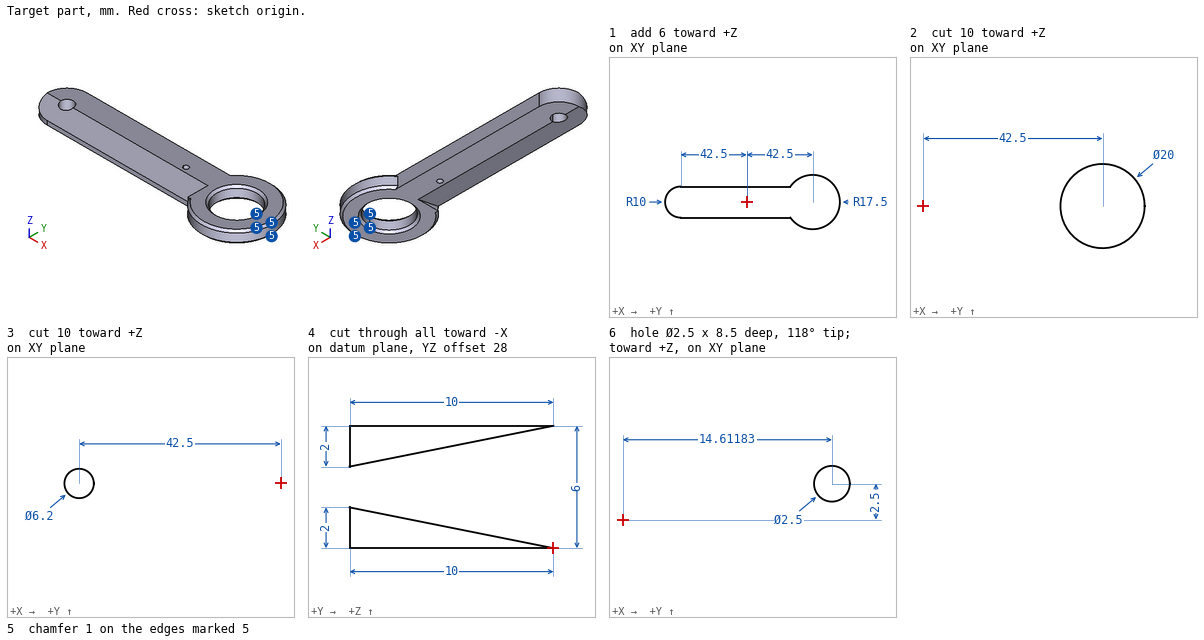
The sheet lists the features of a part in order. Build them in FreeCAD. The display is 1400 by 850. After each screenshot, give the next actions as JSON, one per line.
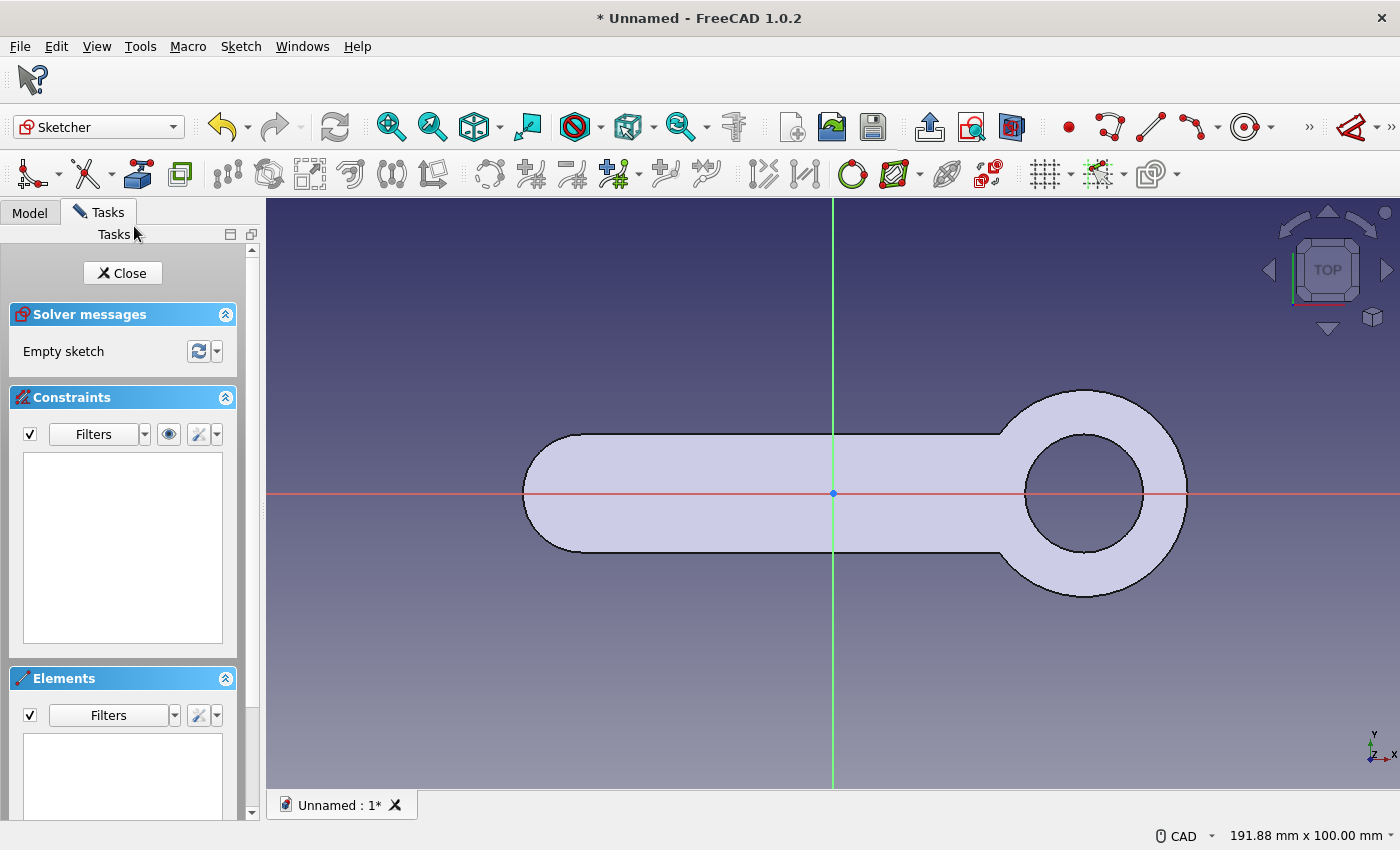
{"action": "scroll", "coordinate": [564, 494], "scroll_direction": "up", "scroll_amount": 12}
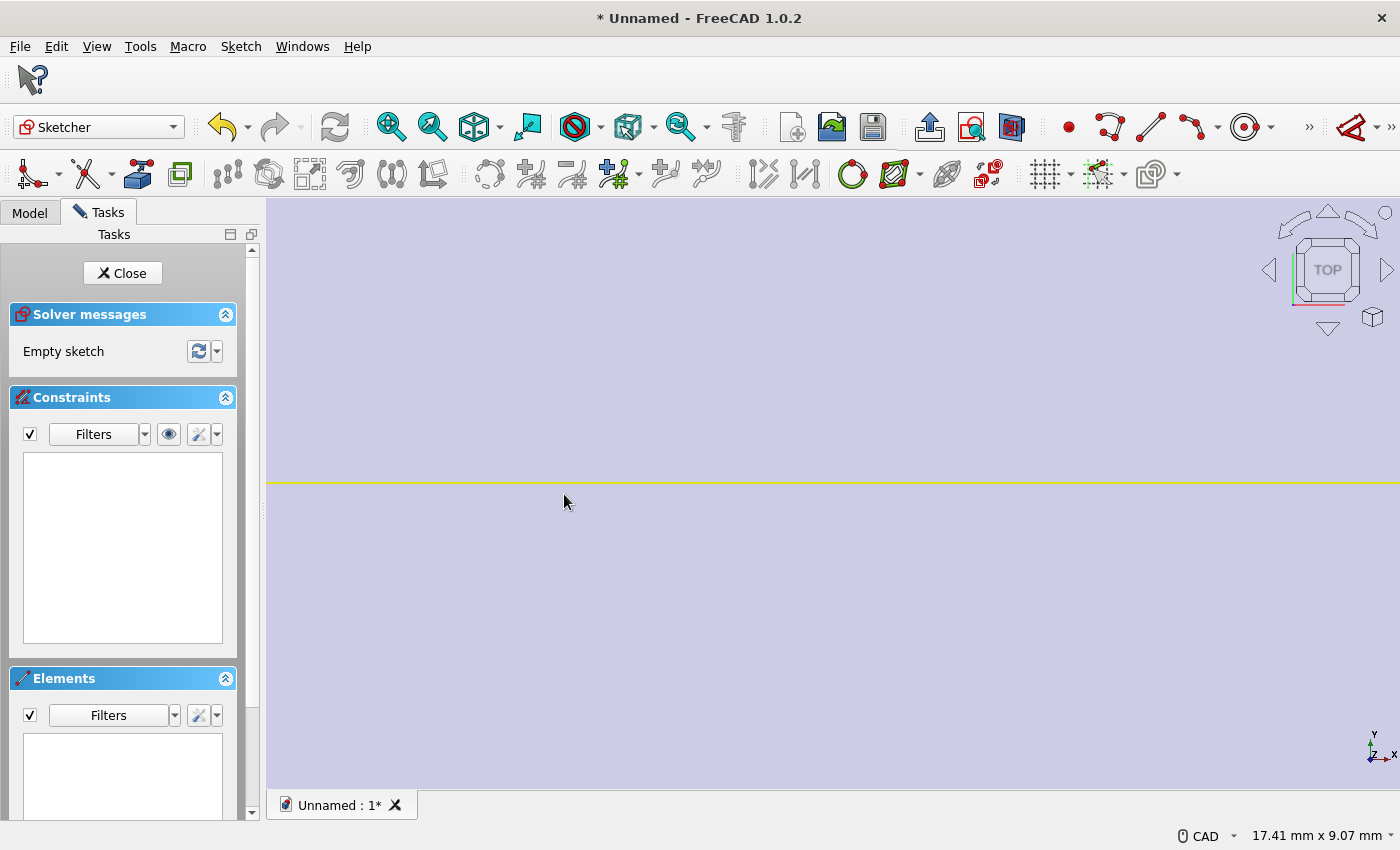
{"action": "key", "text": "g c"}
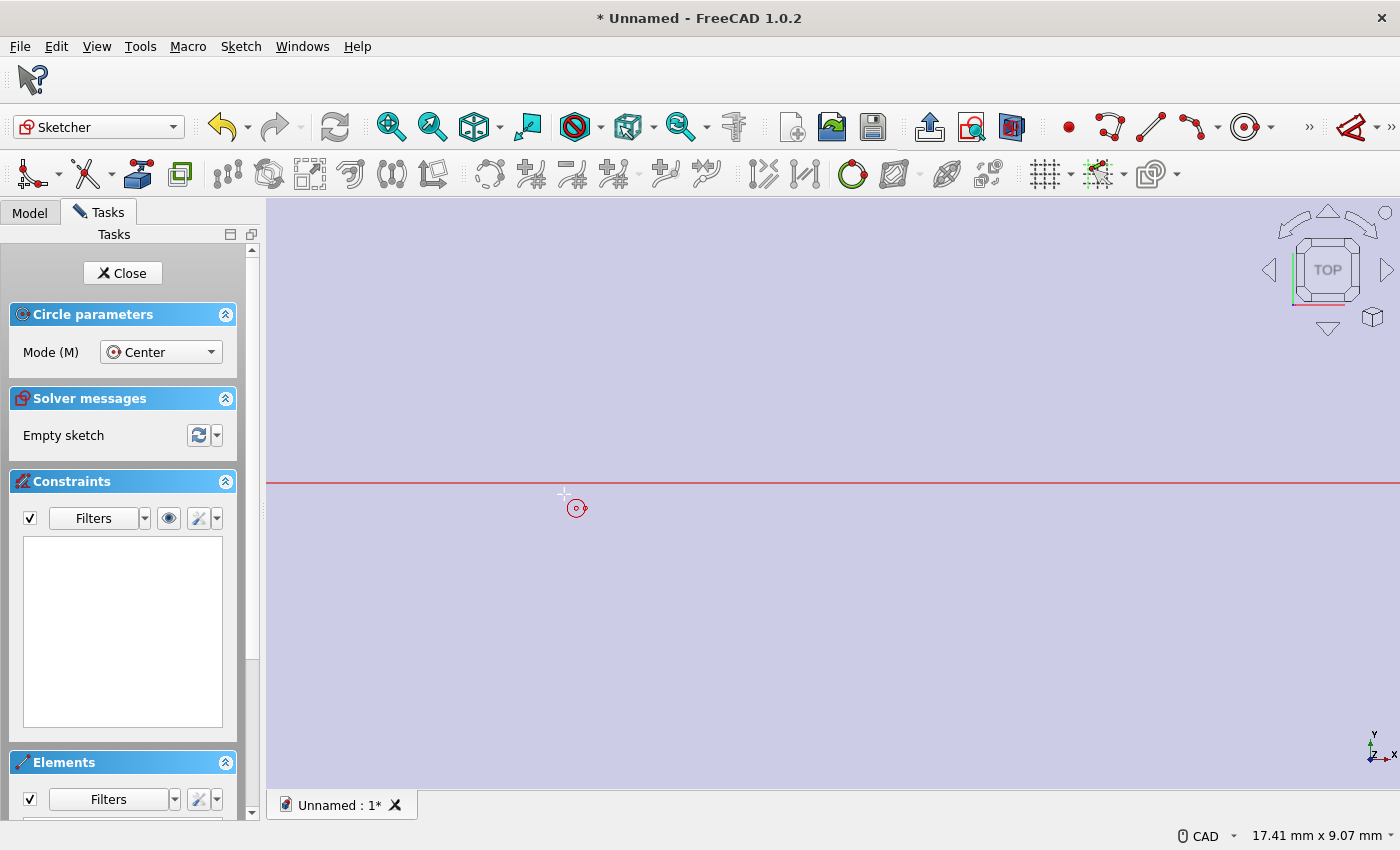
{"action": "left_click", "coordinate": [758, 483]}
{"action": "left_click", "coordinate": [901, 341]}
{"action": "key", "text": "Escape"}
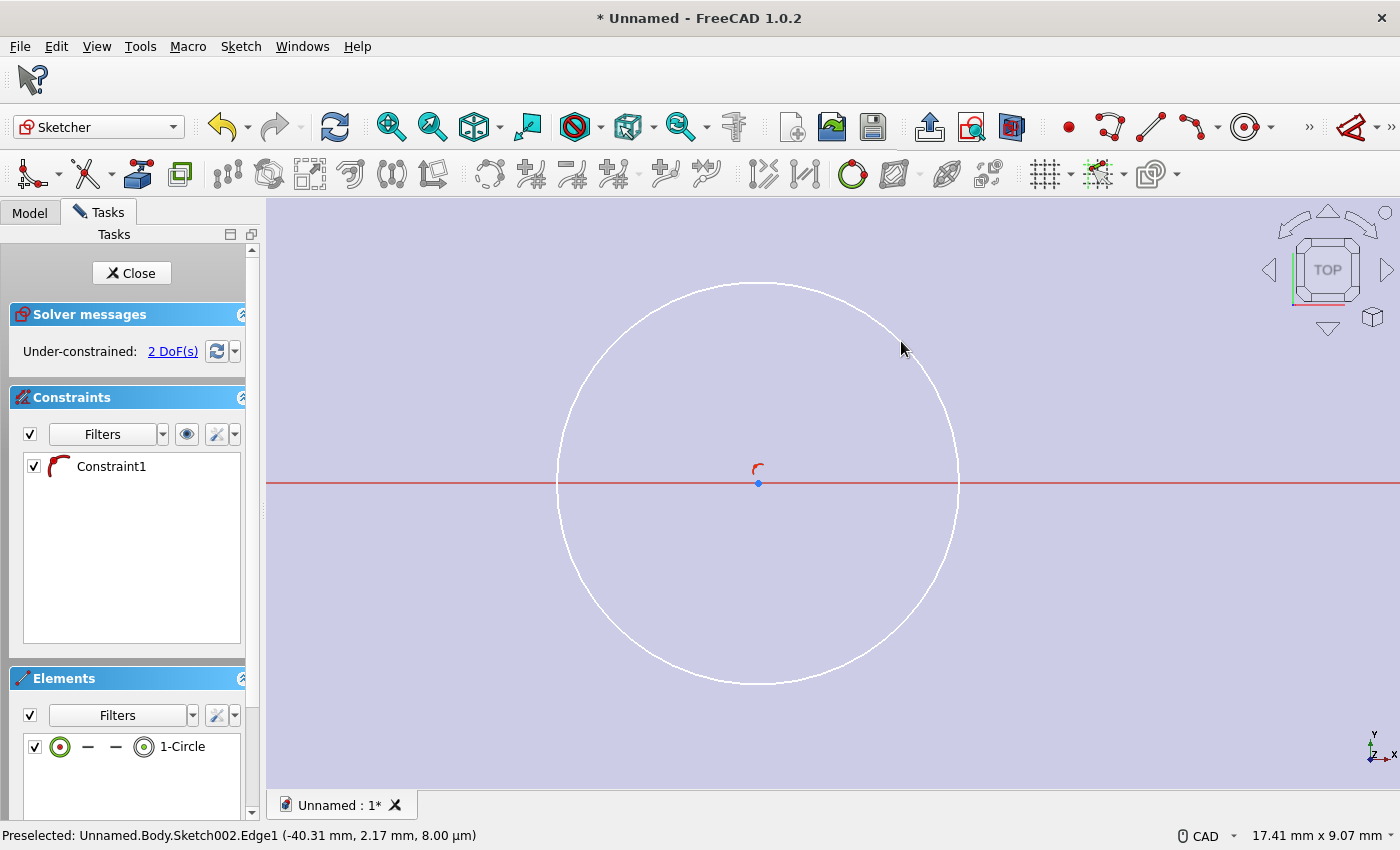
{"action": "key", "text": "d"}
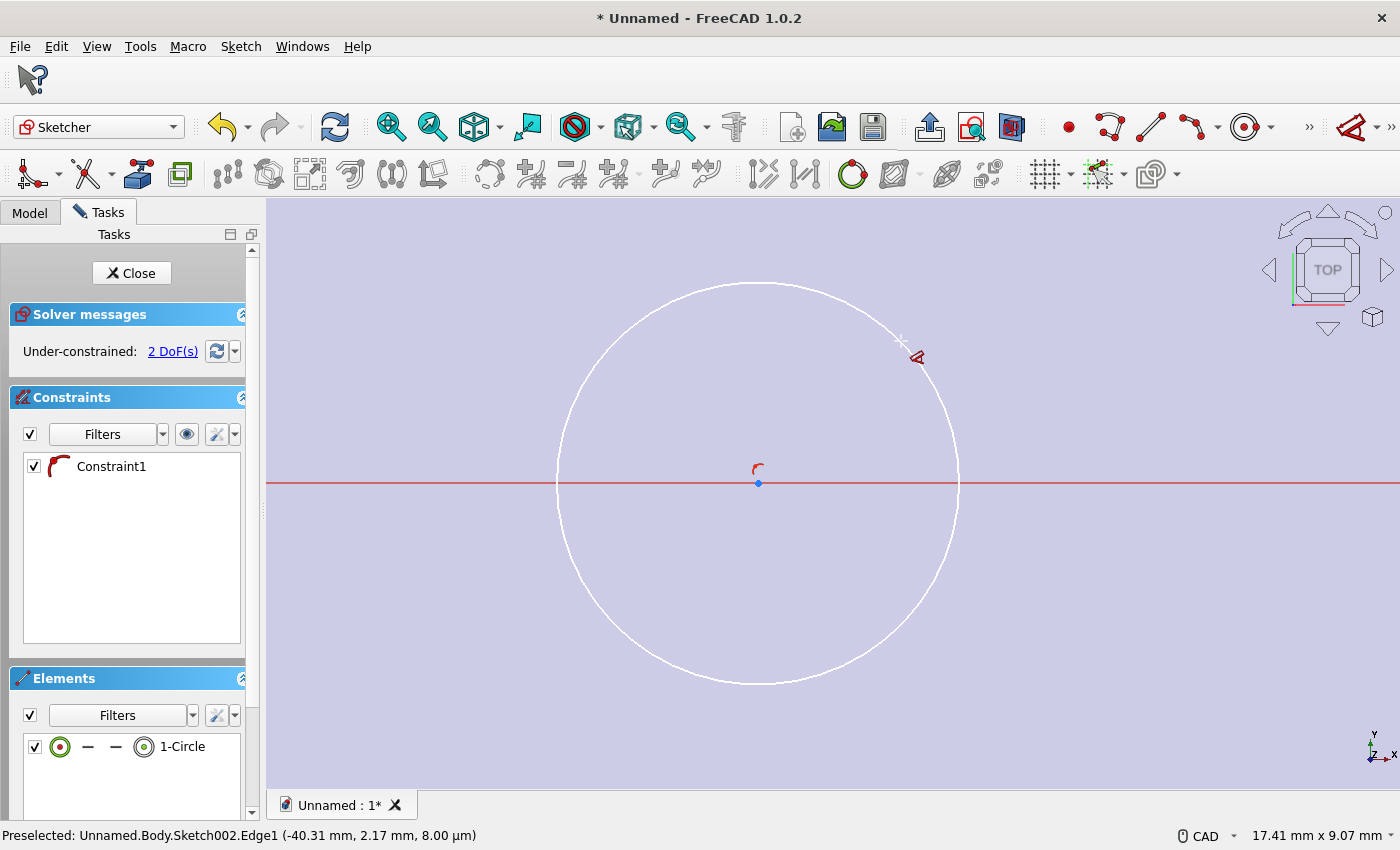
{"action": "left_click", "coordinate": [900, 341]}
{"action": "left_click", "coordinate": [923, 318]}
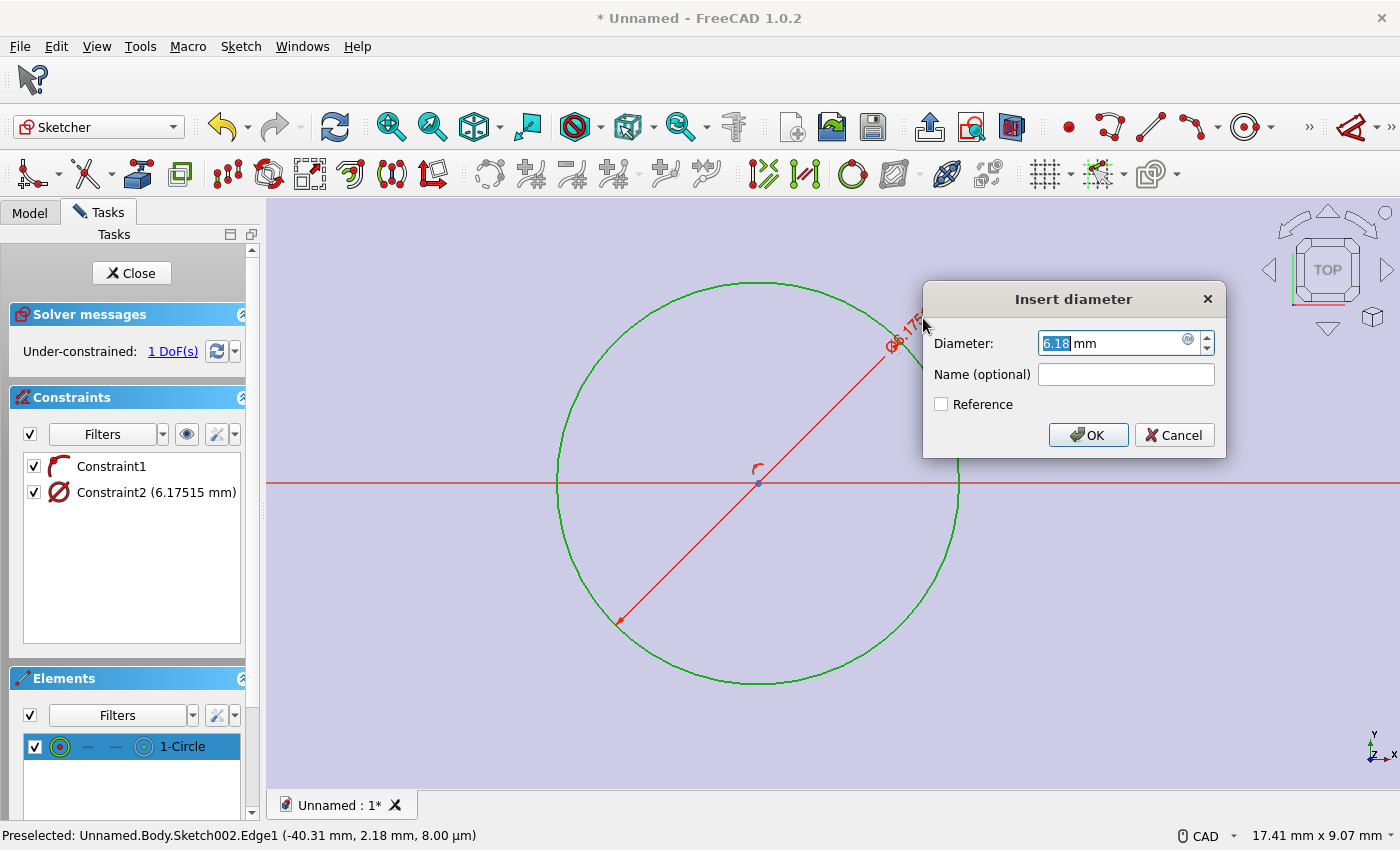
{"action": "type", "text": "6.2"}
{"action": "key", "text": "Return"}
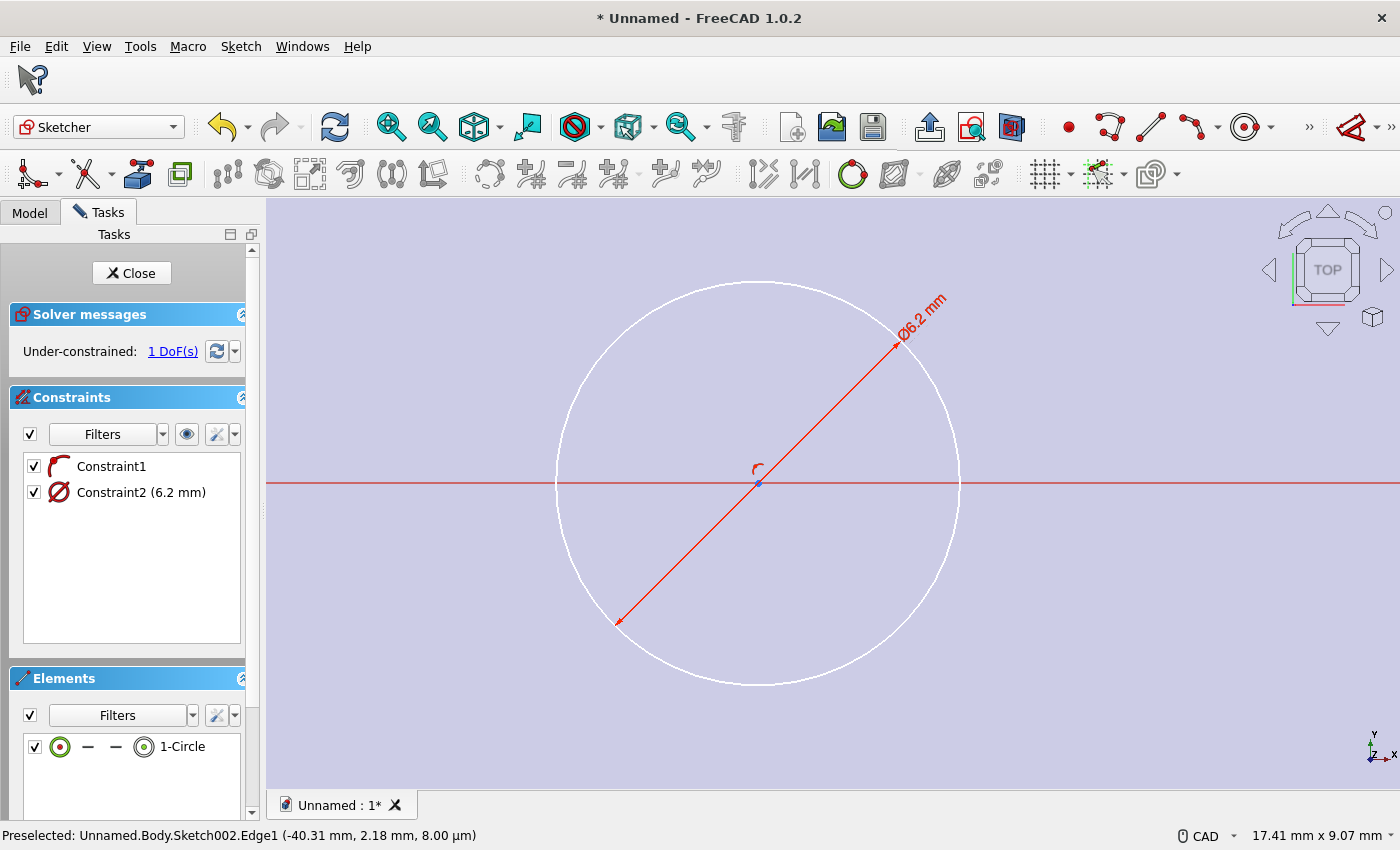
{"action": "left_click", "coordinate": [758, 483]}
{"action": "left_click", "coordinate": [997, 517]}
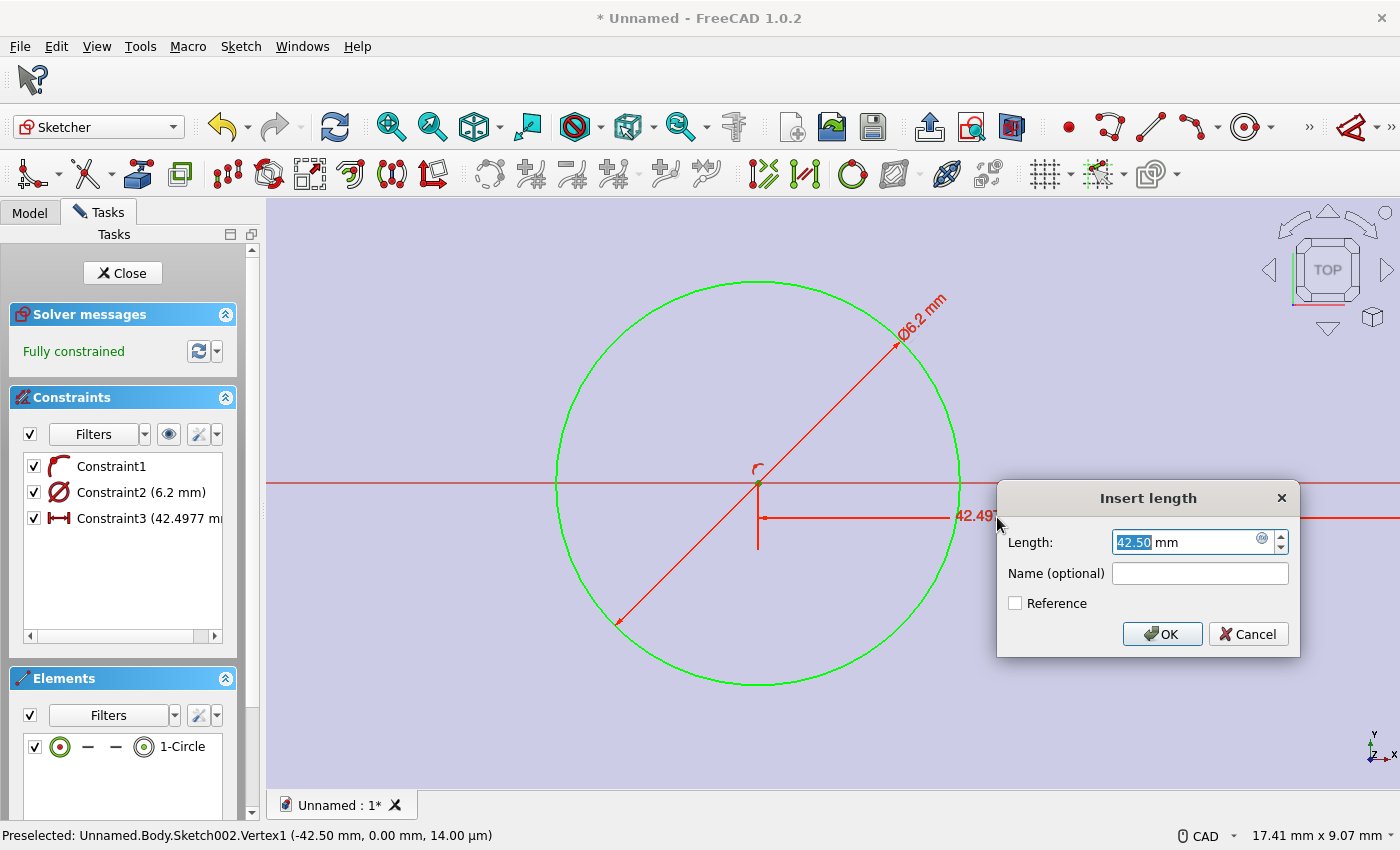
{"action": "type", "text": "42.5"}
{"action": "key", "text": "Return"}
{"action": "key", "text": "Escape"}